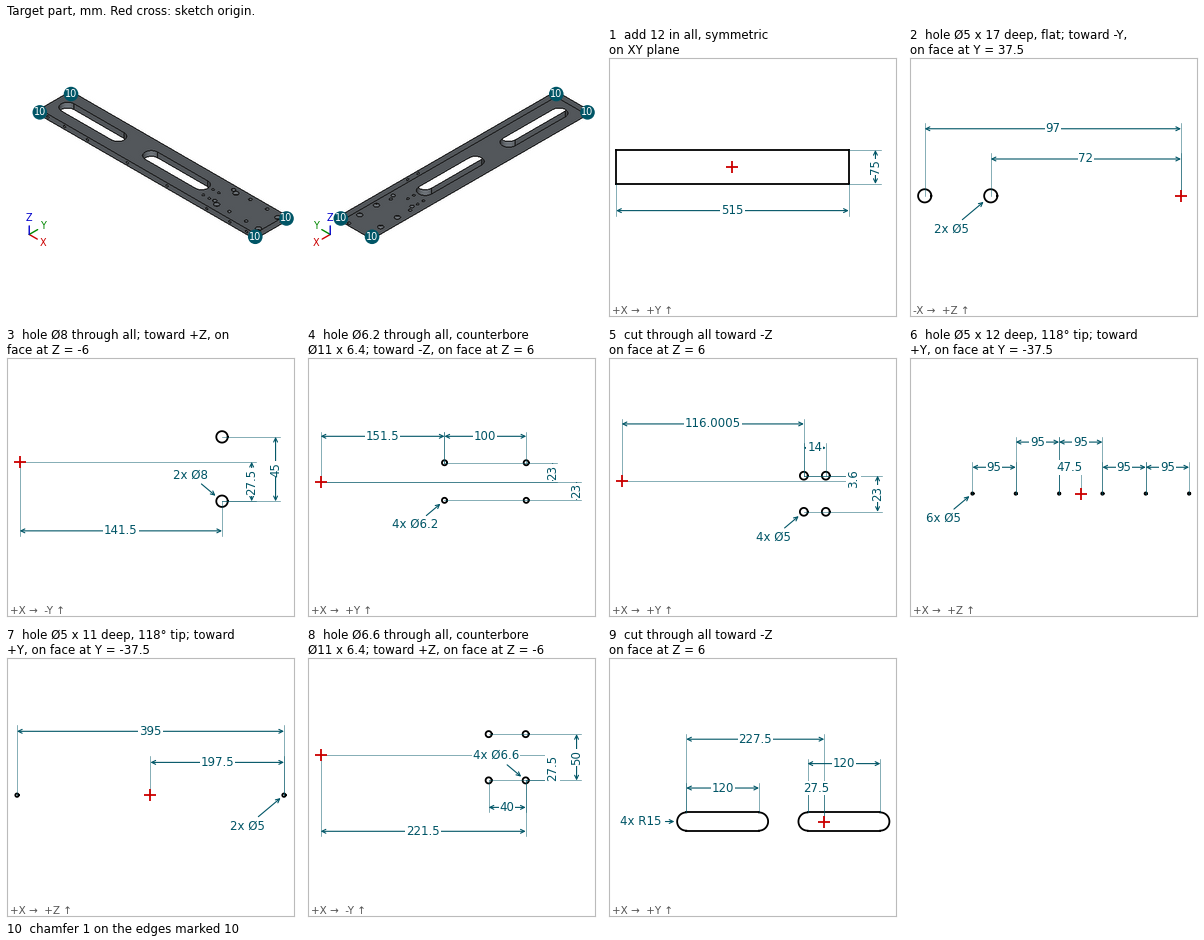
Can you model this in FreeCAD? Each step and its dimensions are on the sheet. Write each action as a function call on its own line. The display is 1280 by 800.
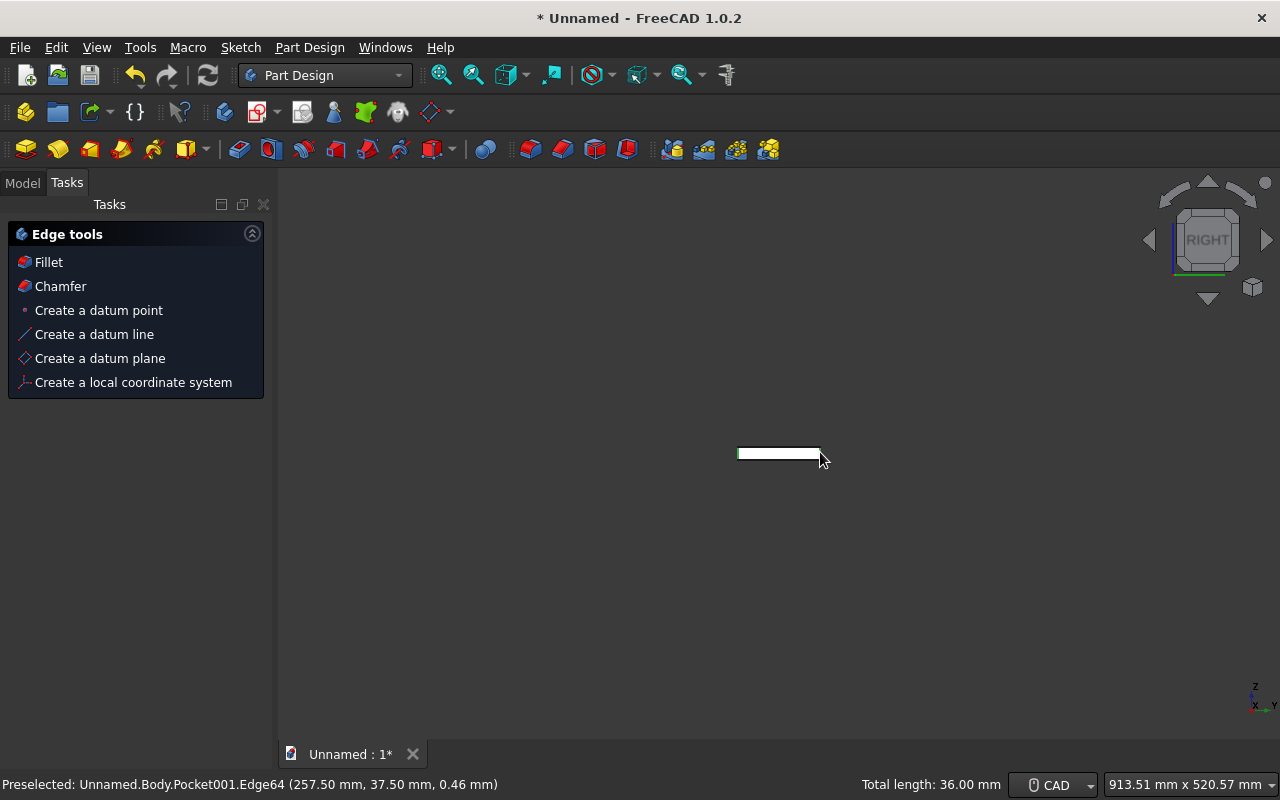
scroll(820, 452, up, 6)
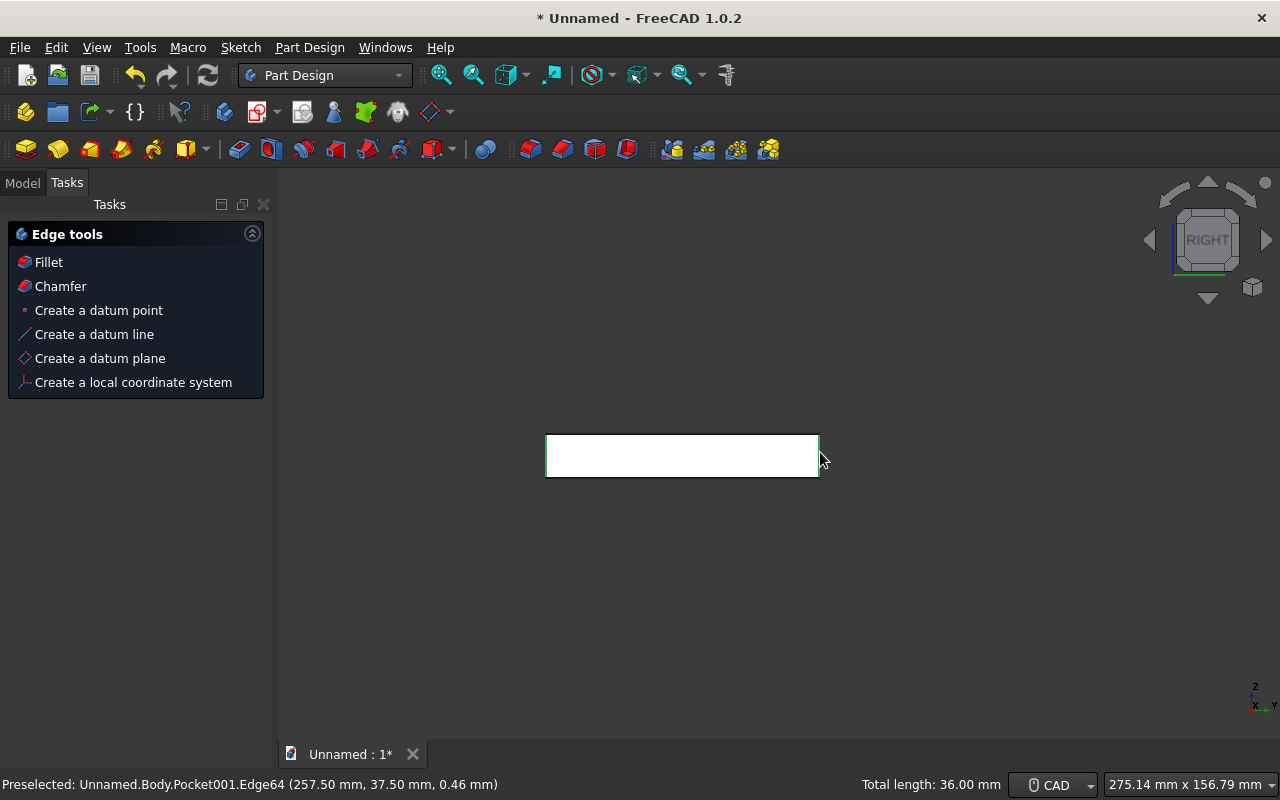
key(v)
key(f)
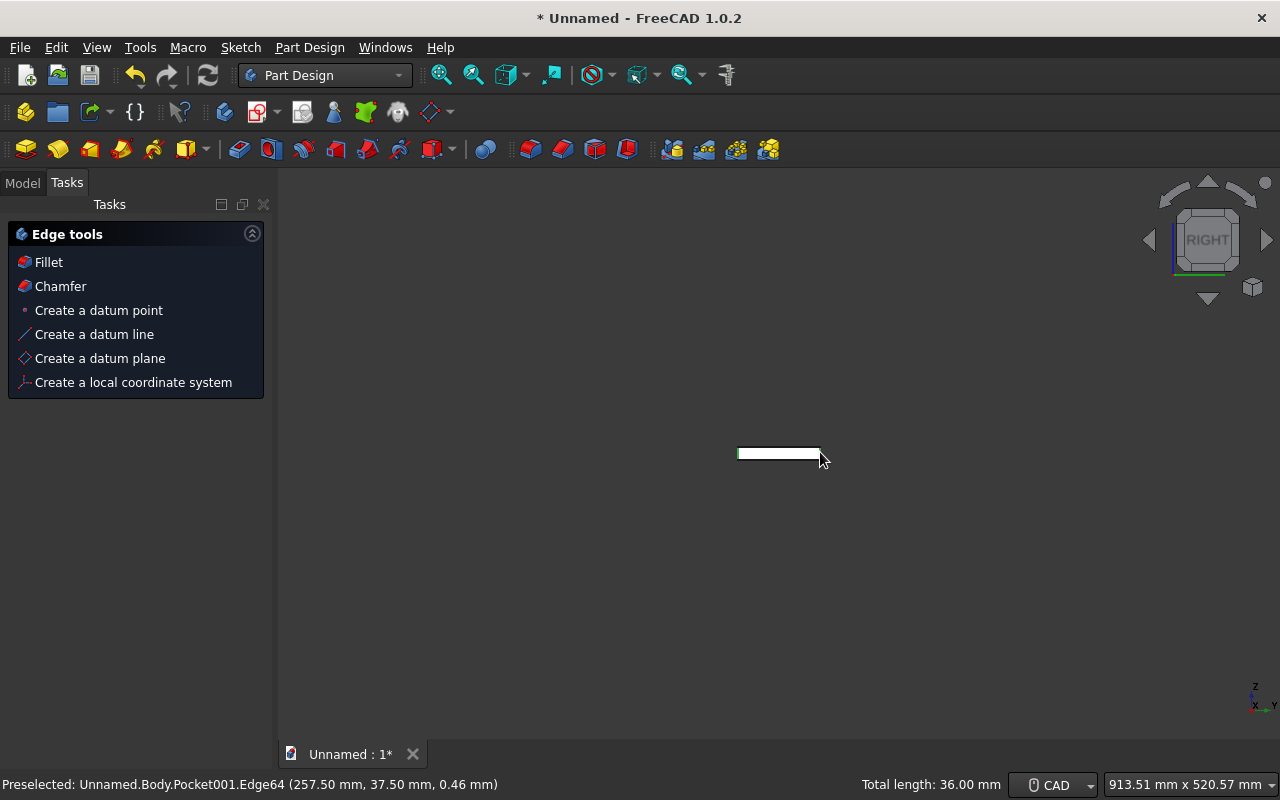
key(5)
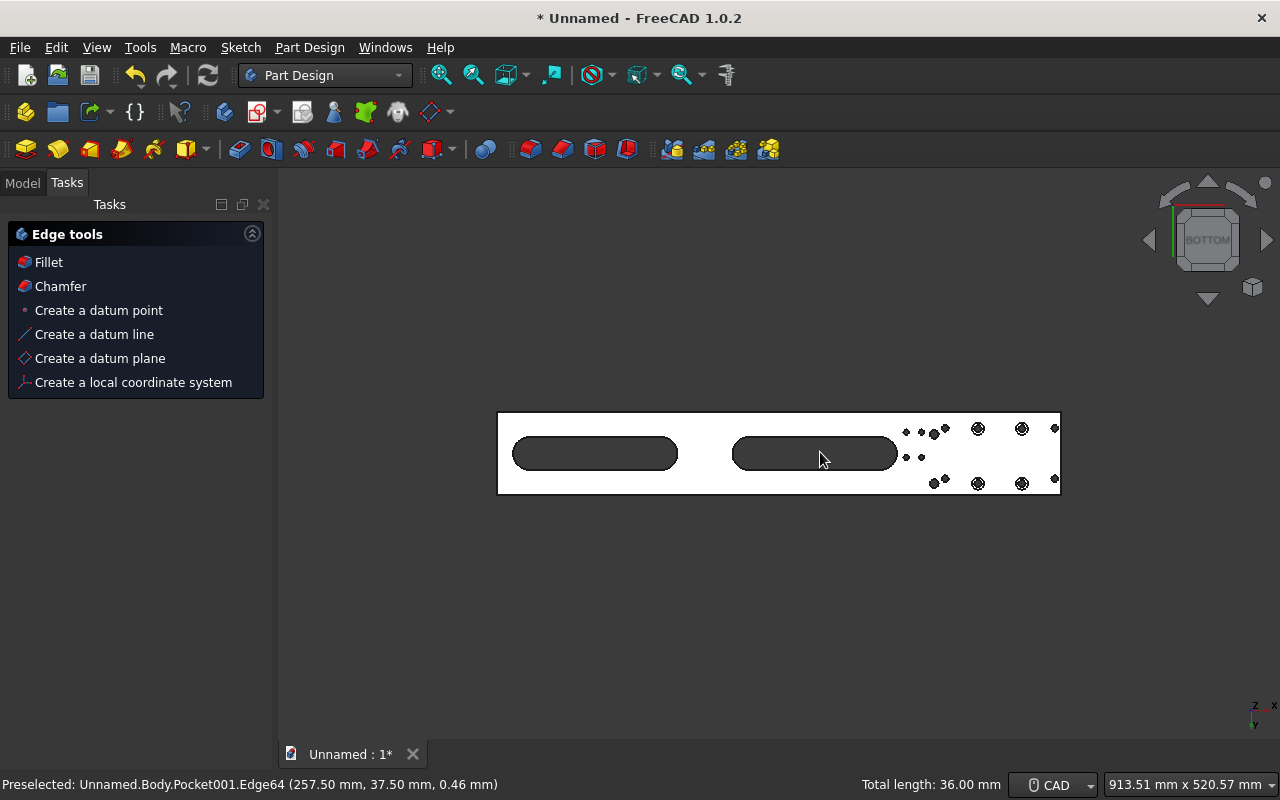
scroll(497, 494, up, 6)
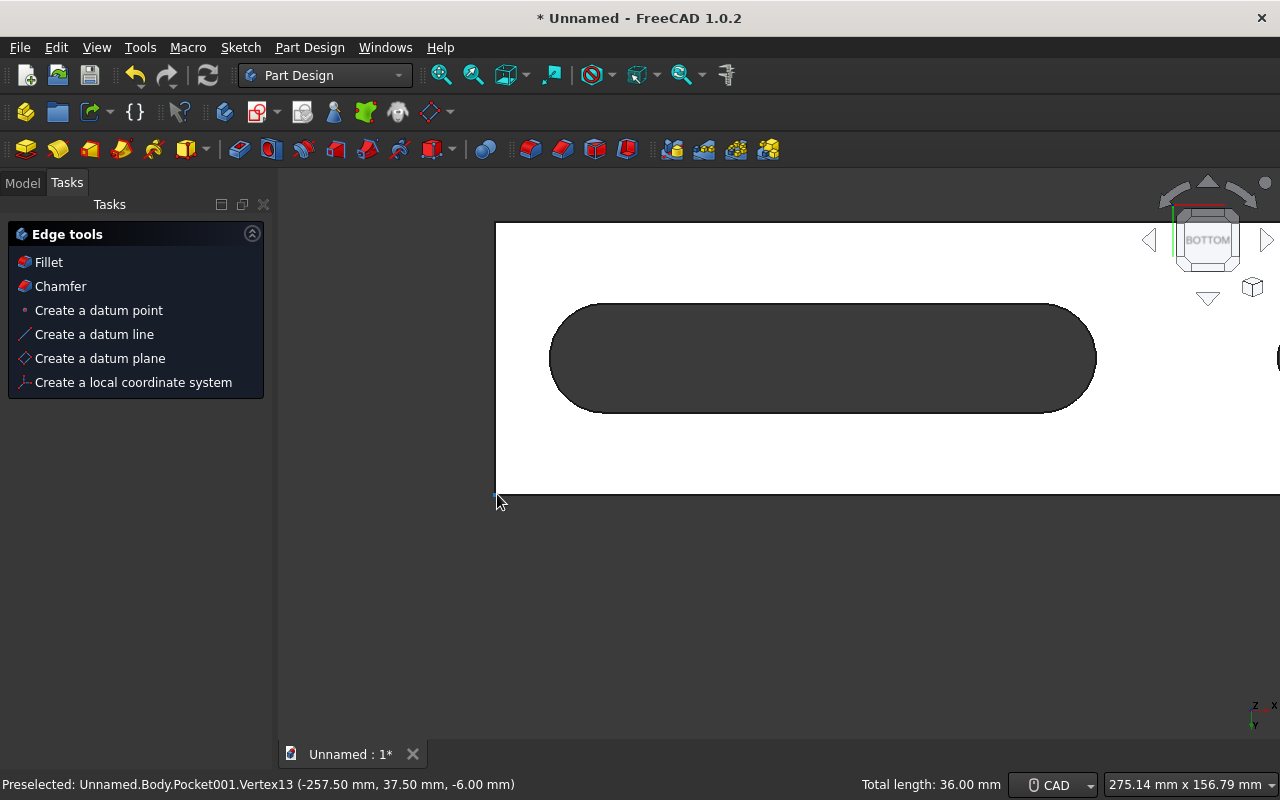
key(v)
key(f)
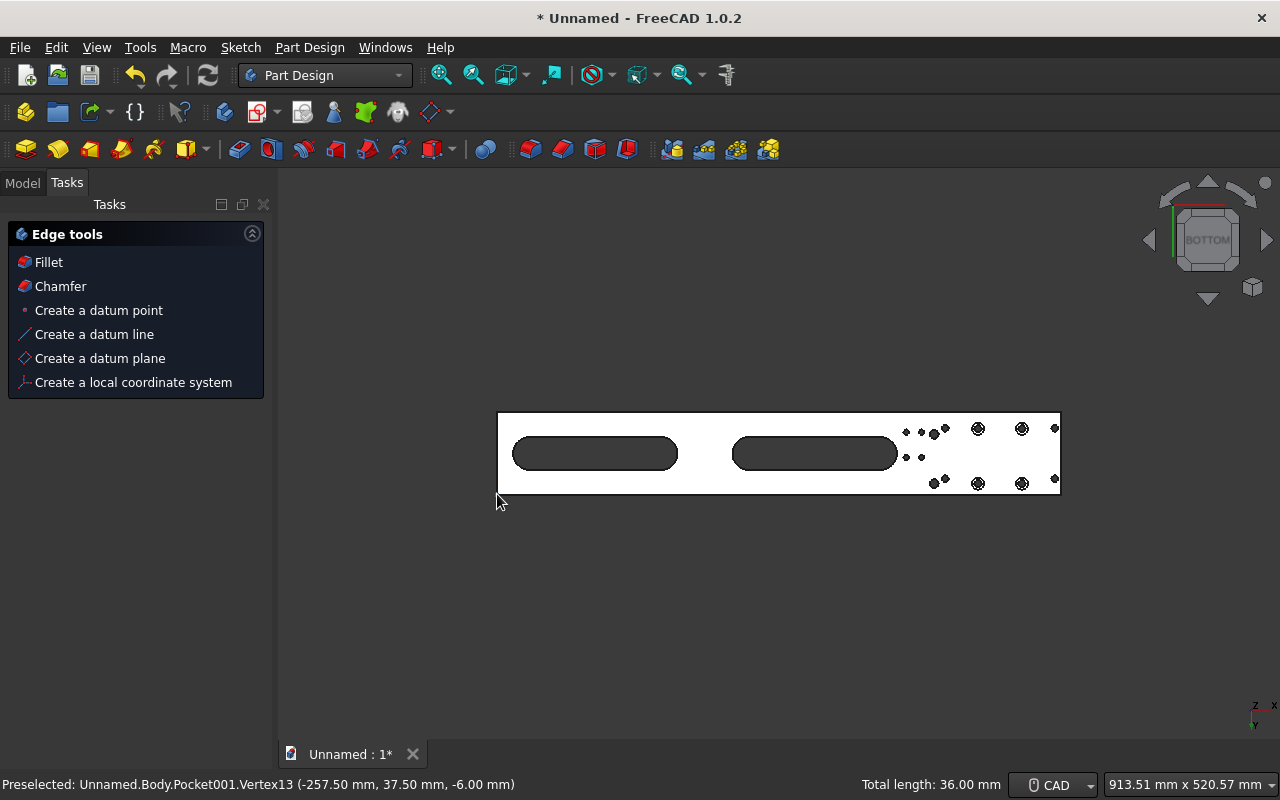
key(4)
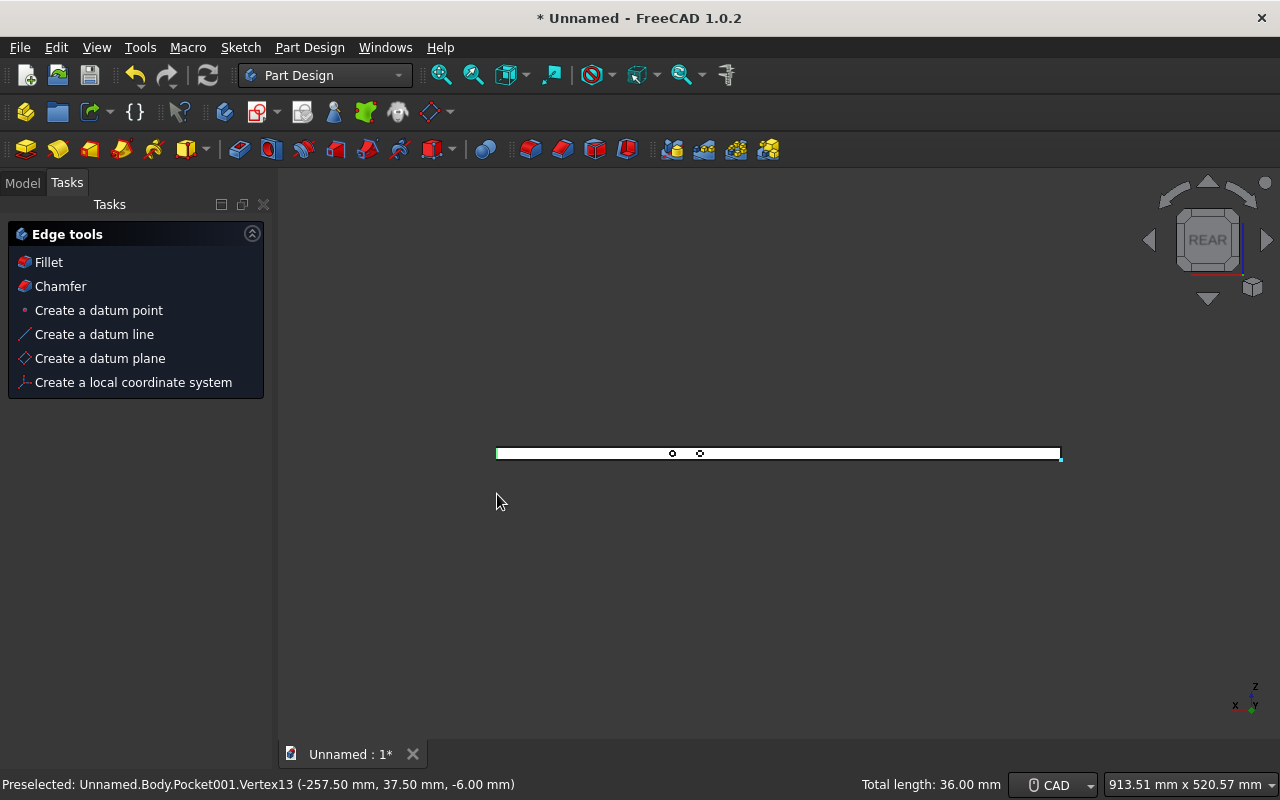
click(1061, 452, ctrl)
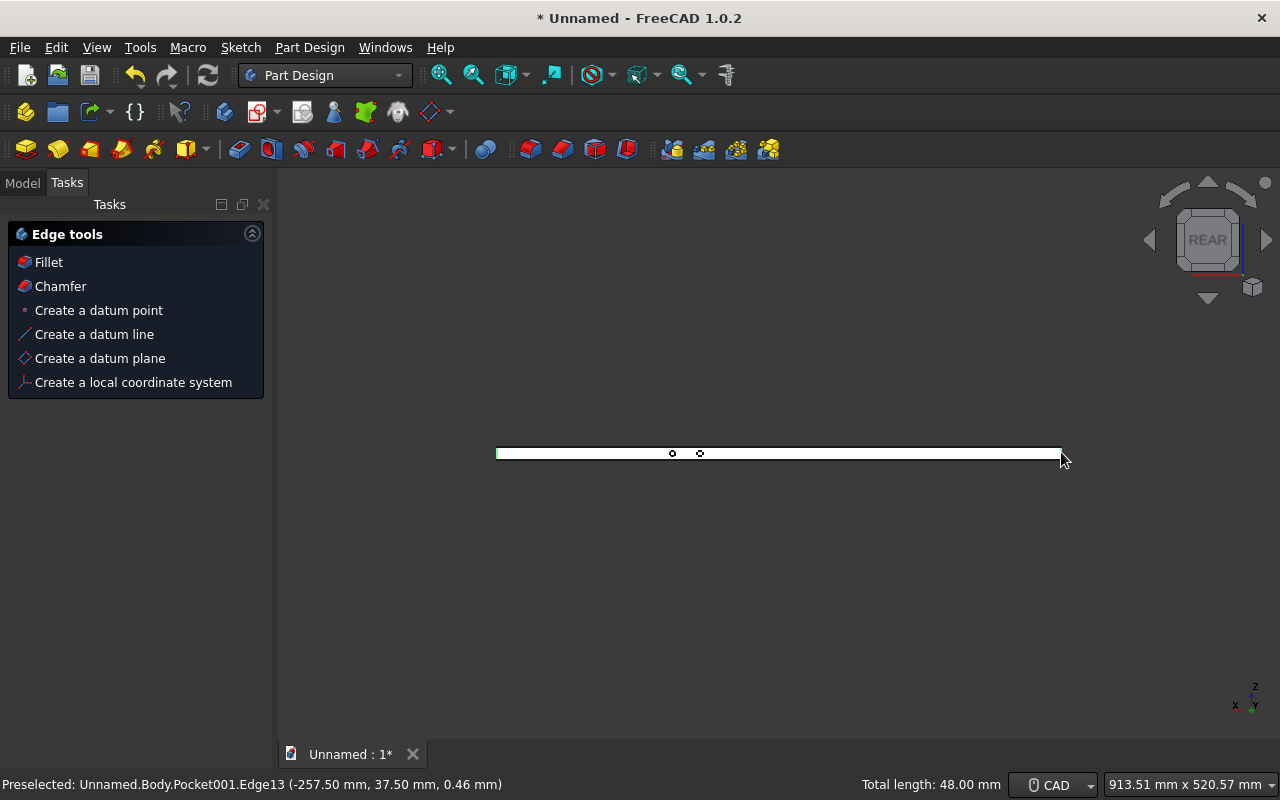
click(564, 150)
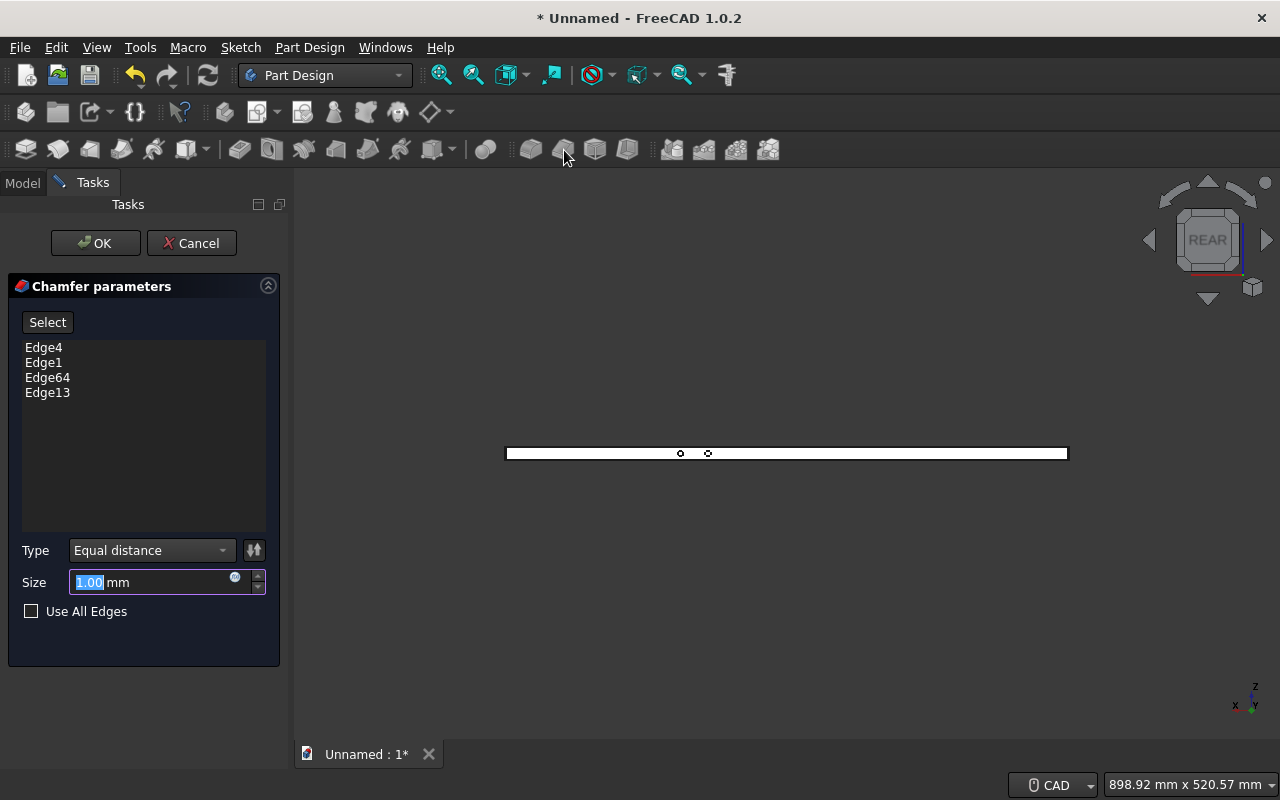
text(1)
key(Tab)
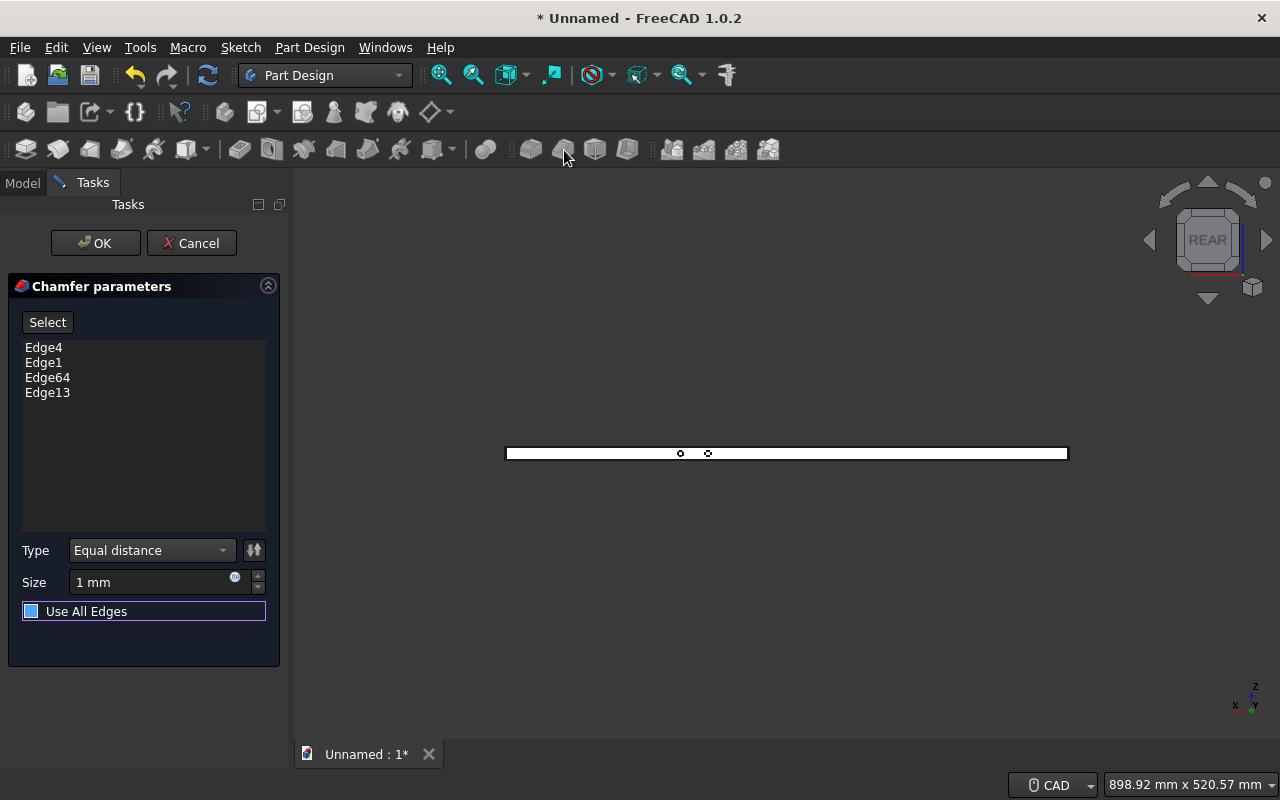
click(96, 243)